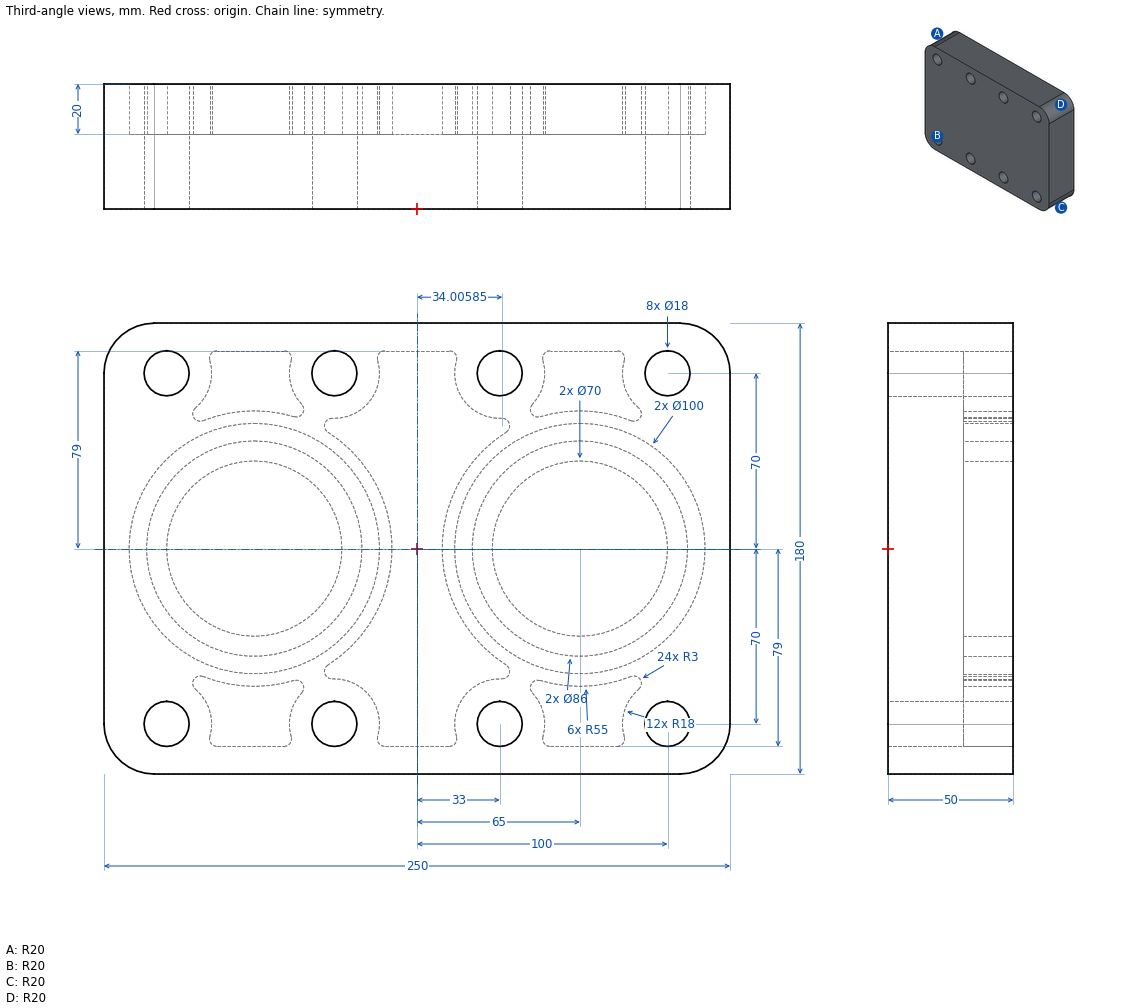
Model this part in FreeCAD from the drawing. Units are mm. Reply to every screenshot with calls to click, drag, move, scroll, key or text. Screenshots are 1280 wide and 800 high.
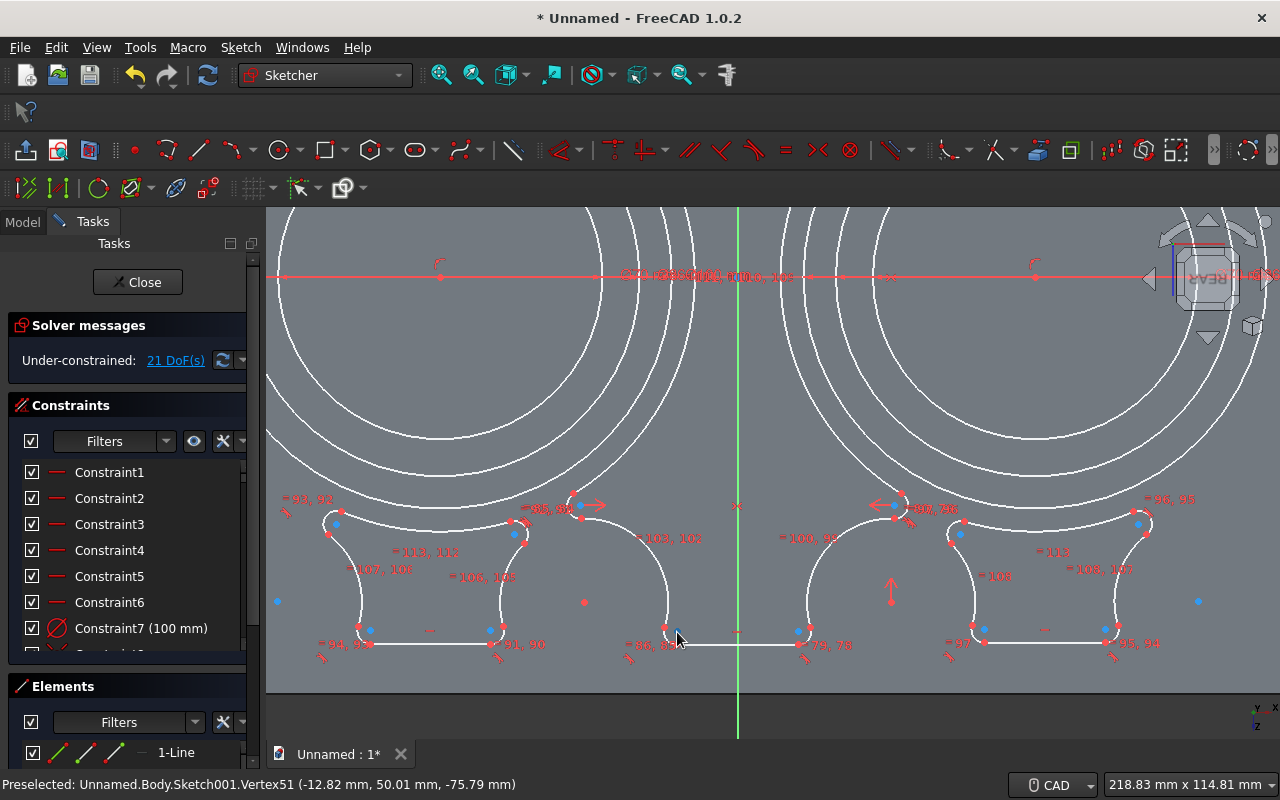
click(677, 632)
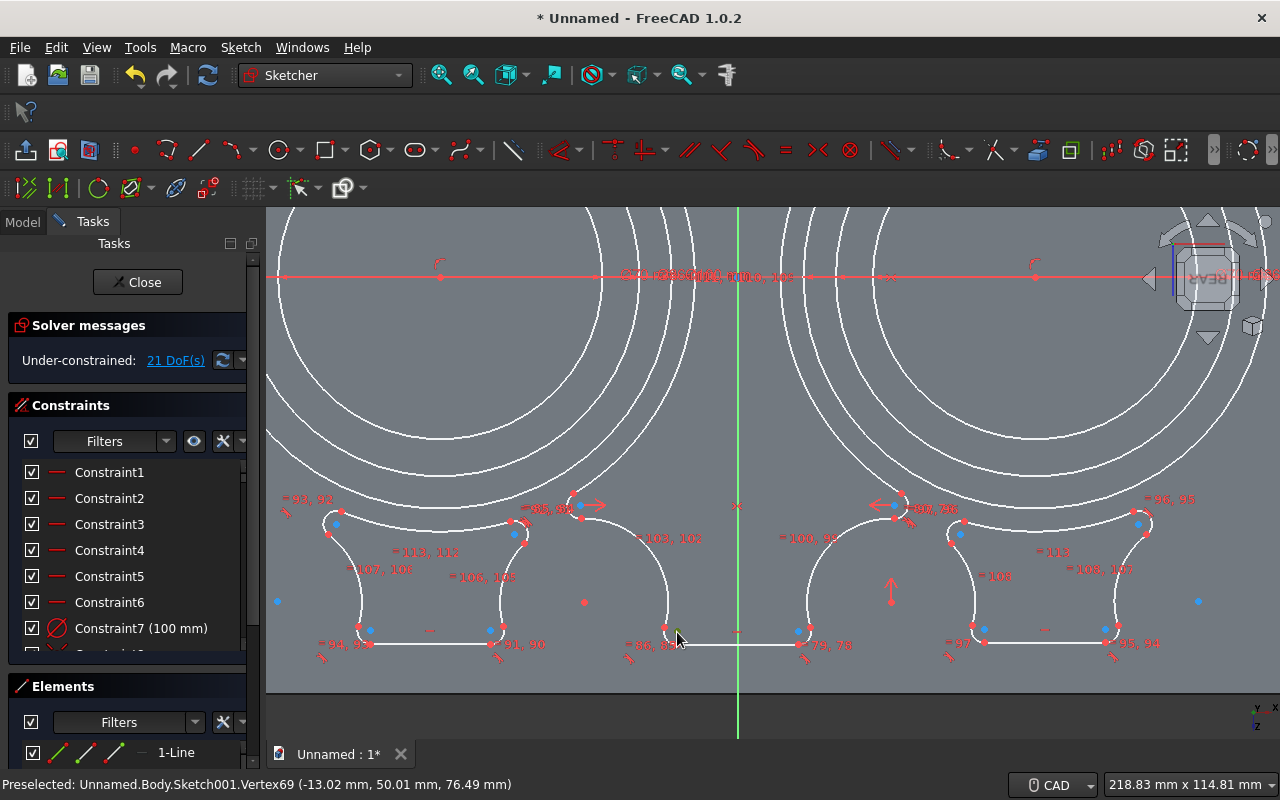
click(353, 277)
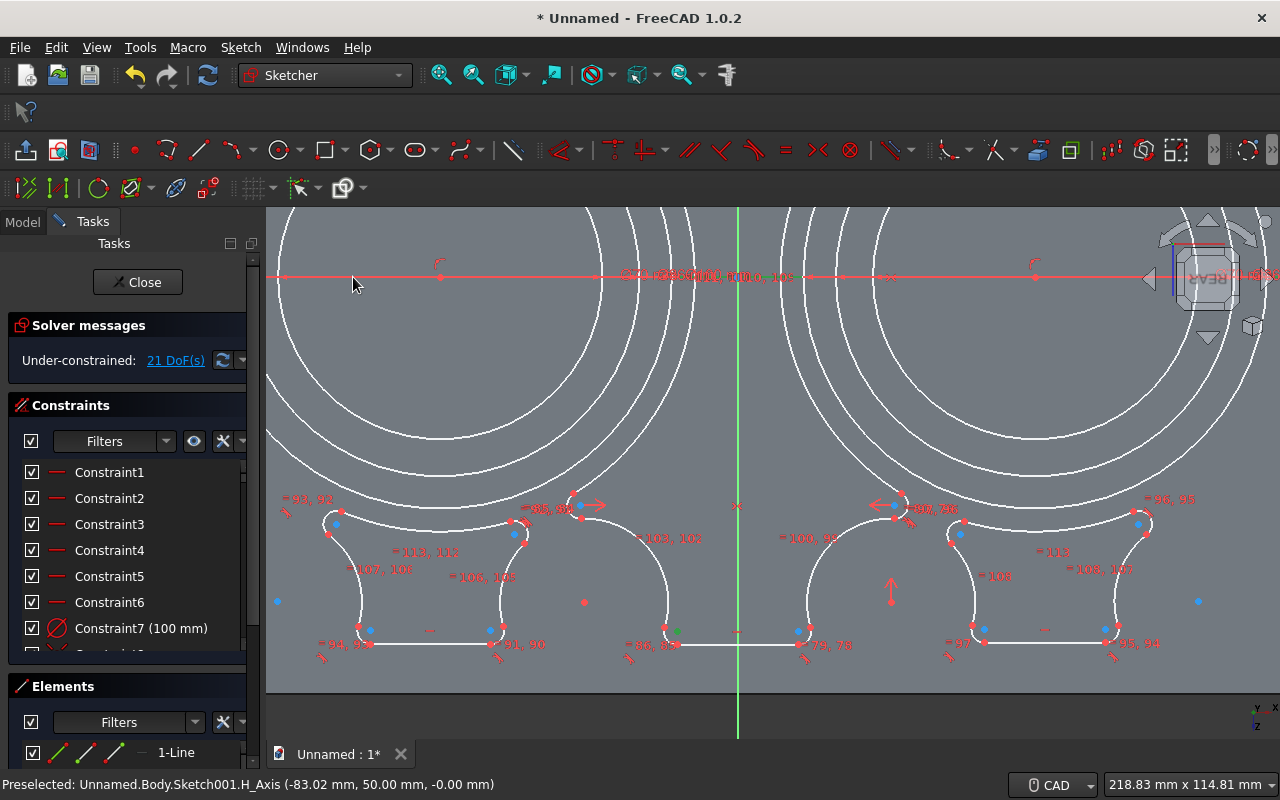
click(818, 150)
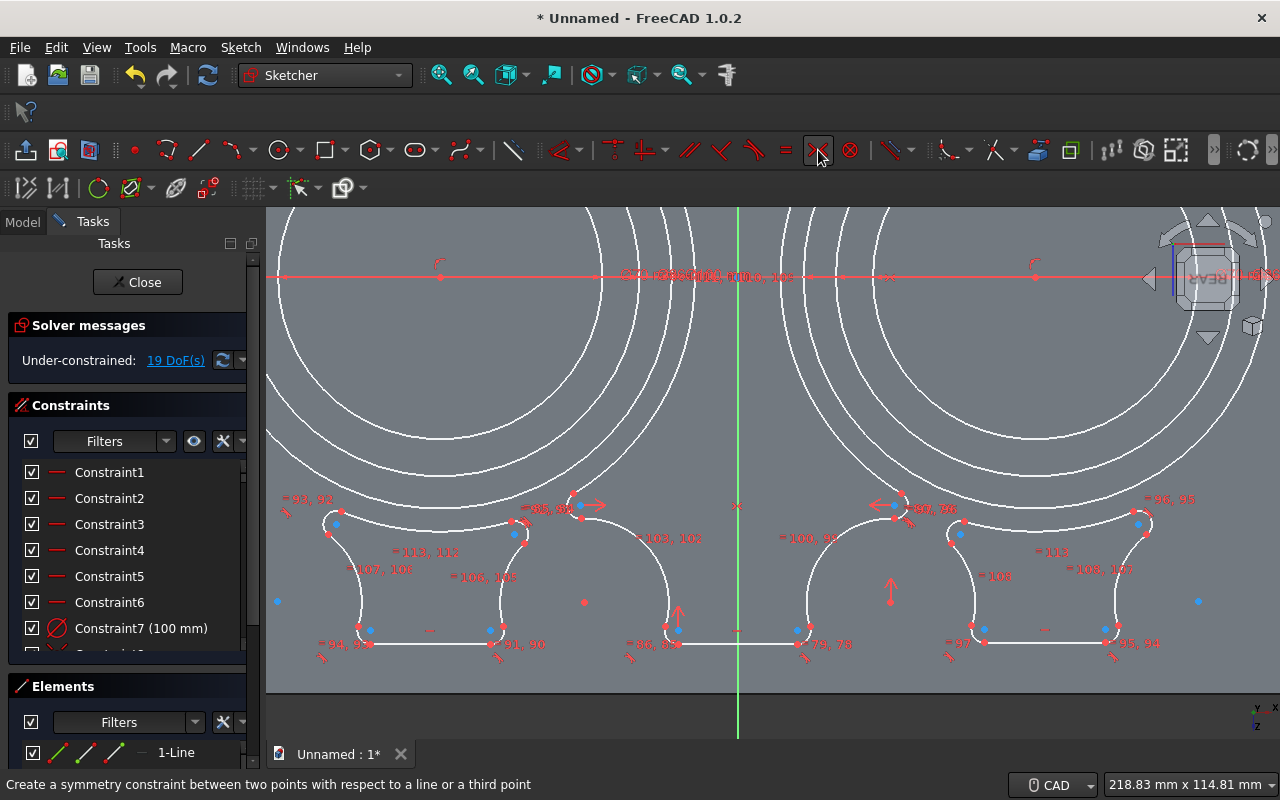
scroll(677, 633, down, 4)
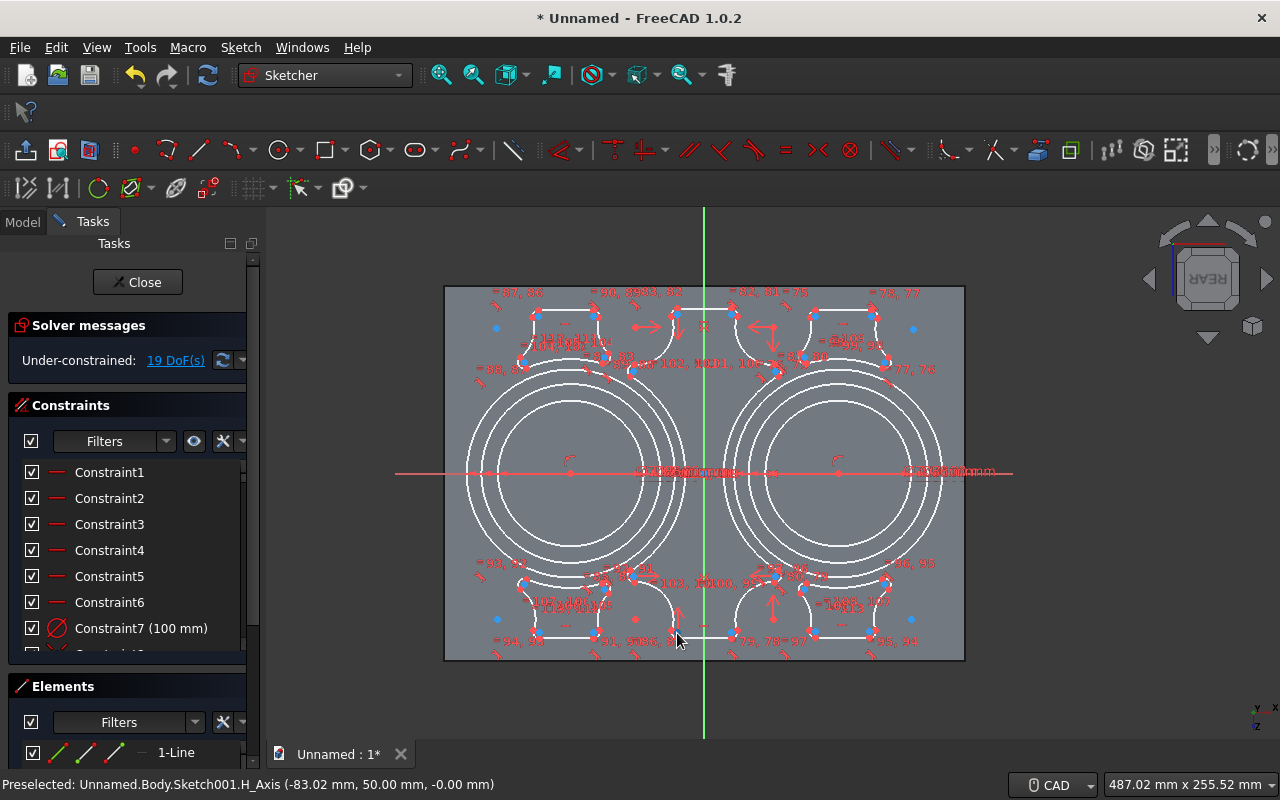
scroll(871, 316, up, 4)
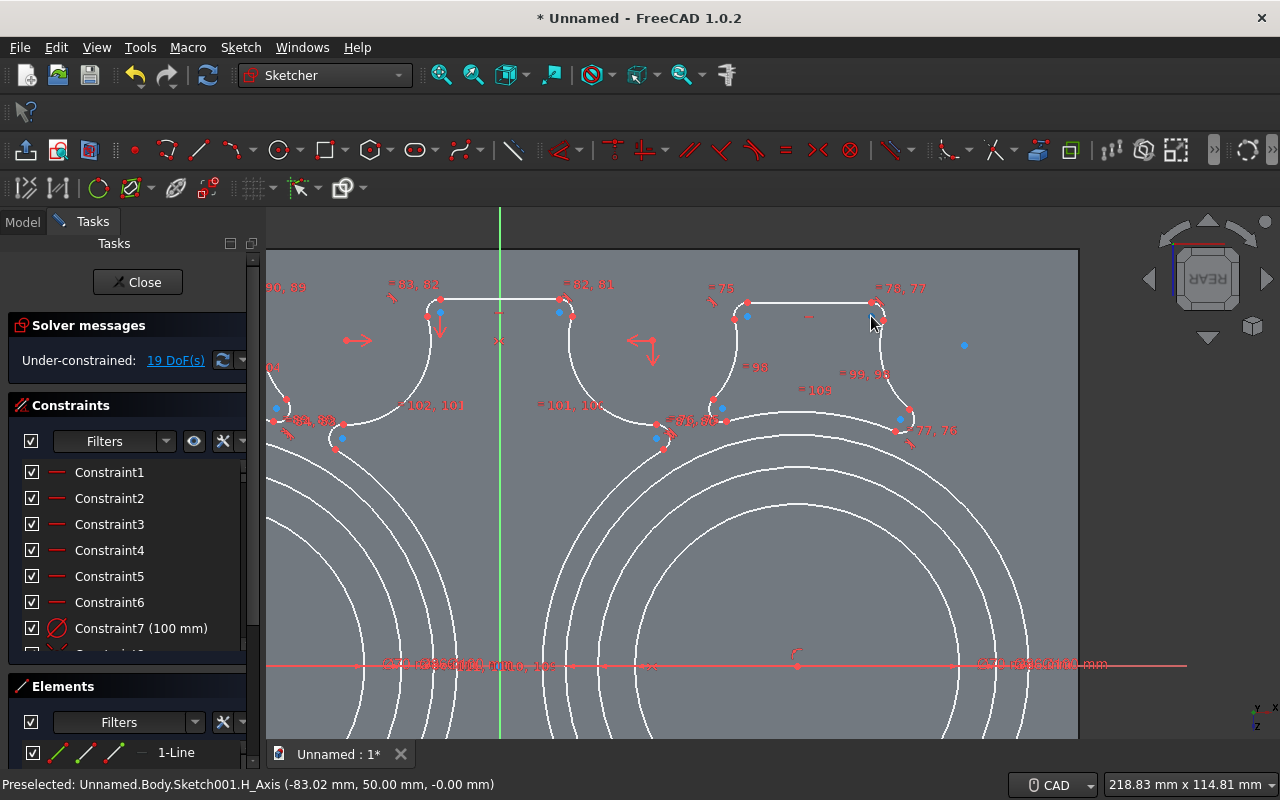
click(871, 316)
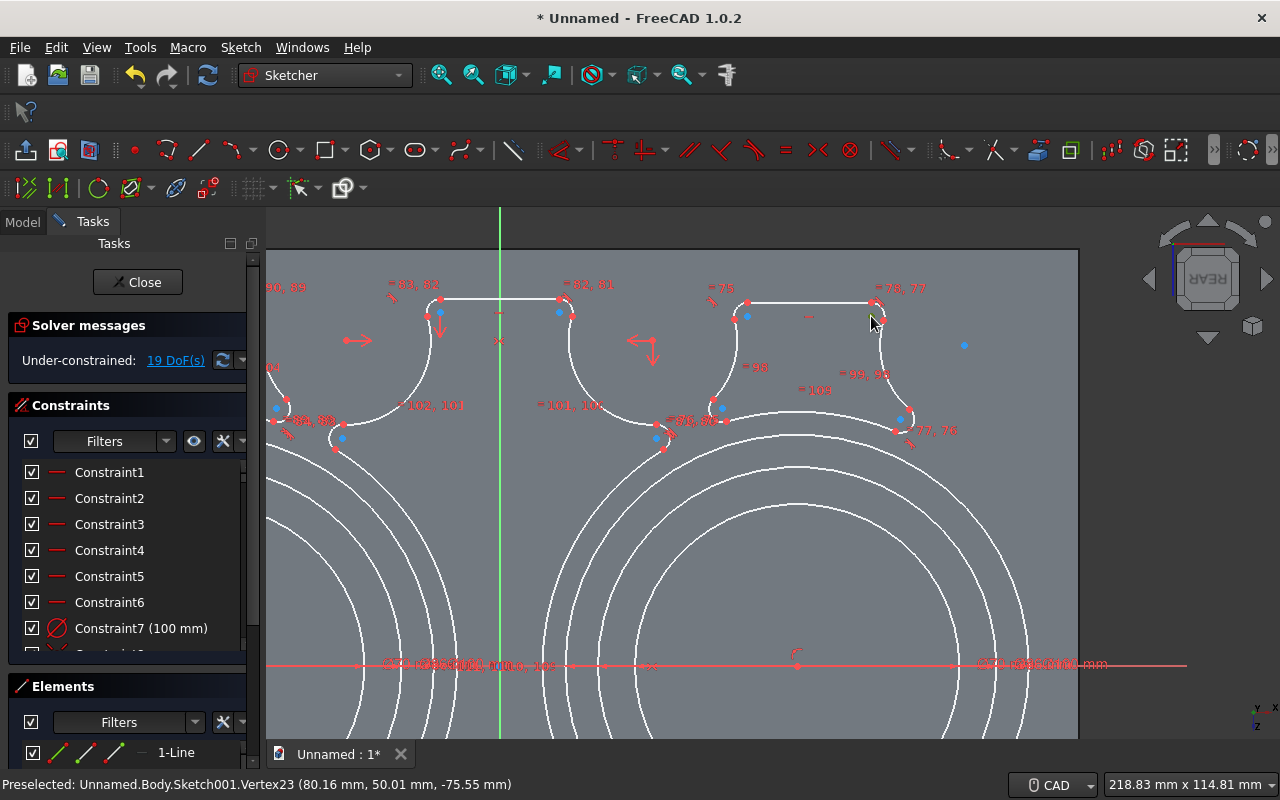
scroll(872, 315, down, 4)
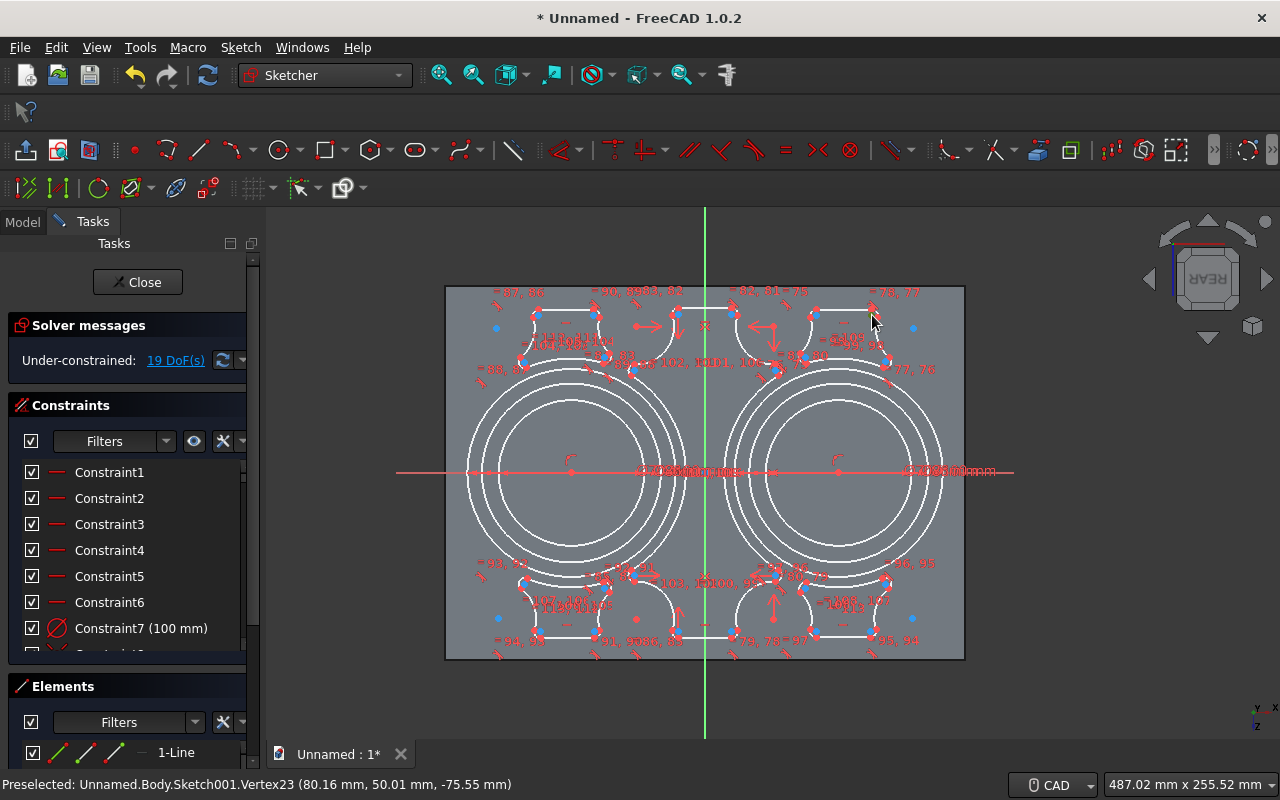
scroll(539, 316, up, 4)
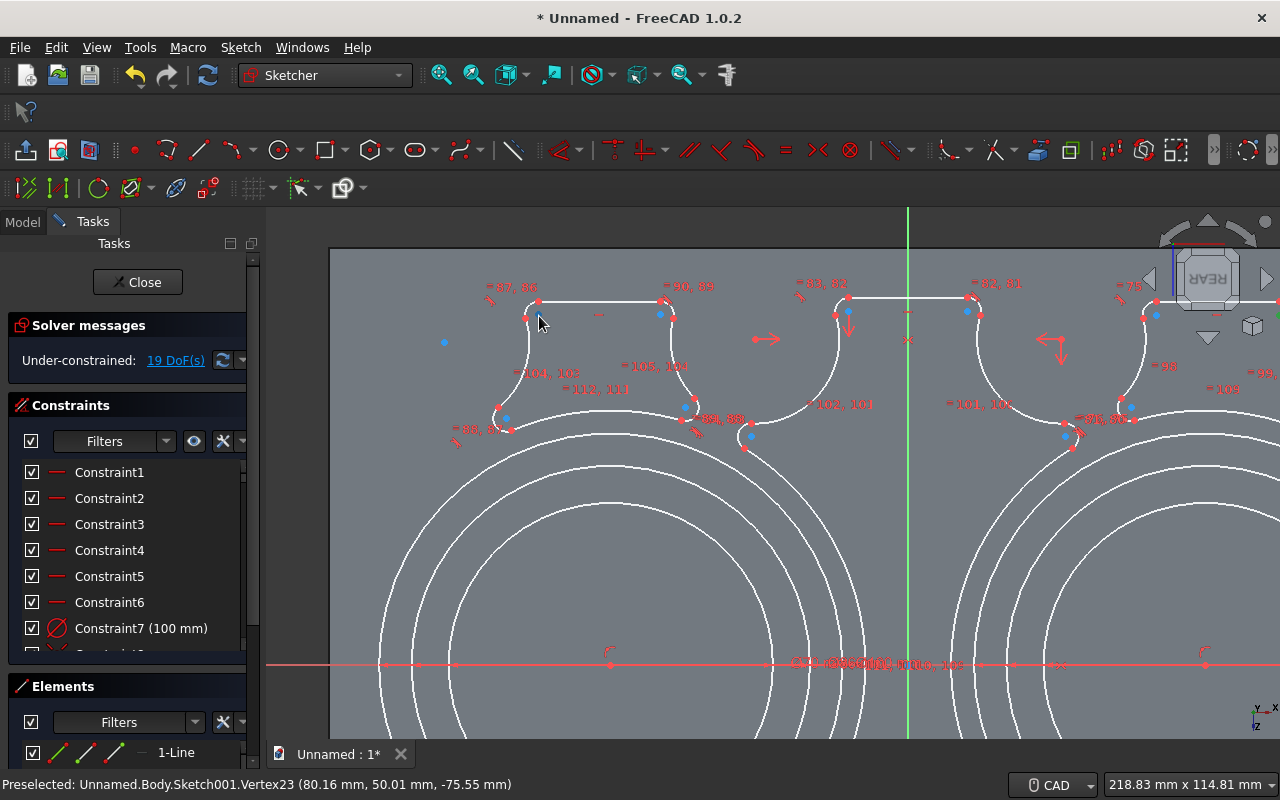
click(539, 315)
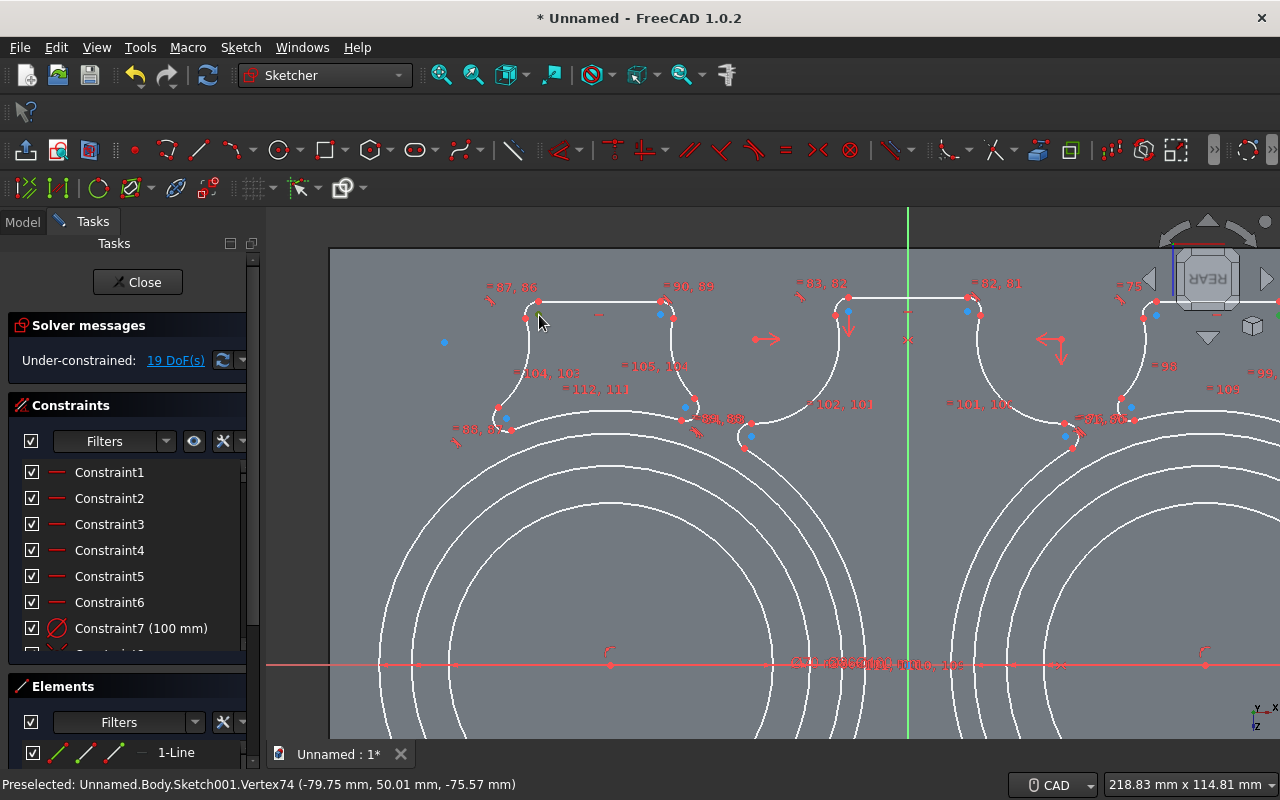
click(908, 609)